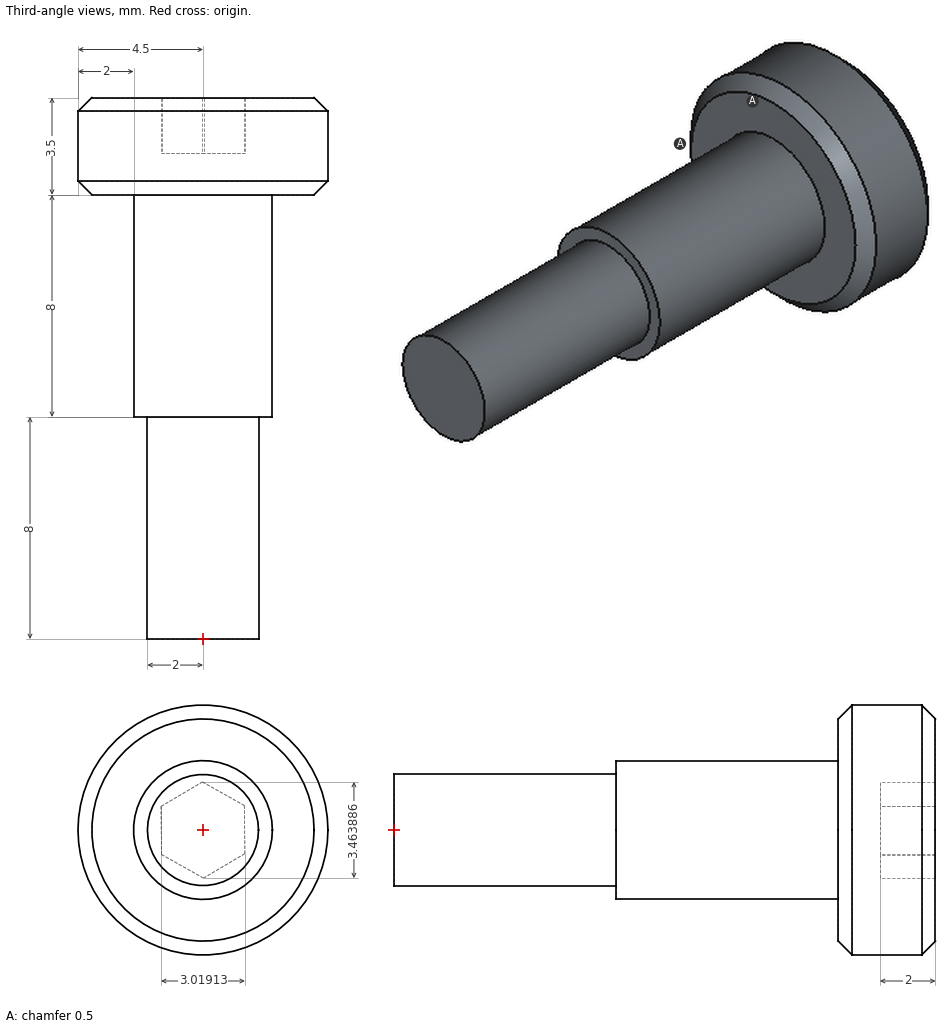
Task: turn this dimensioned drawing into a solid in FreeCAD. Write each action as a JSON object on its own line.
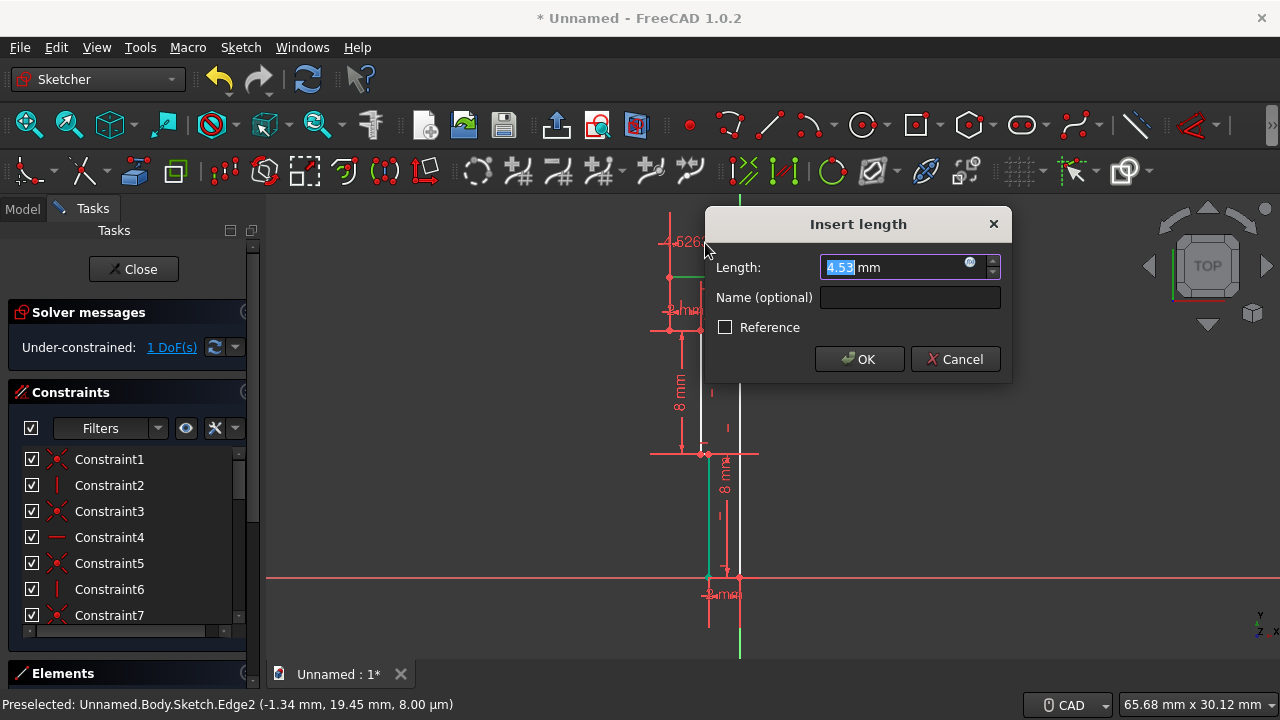
{"action": "type", "text": "4.5"}
{"action": "key", "text": "Return"}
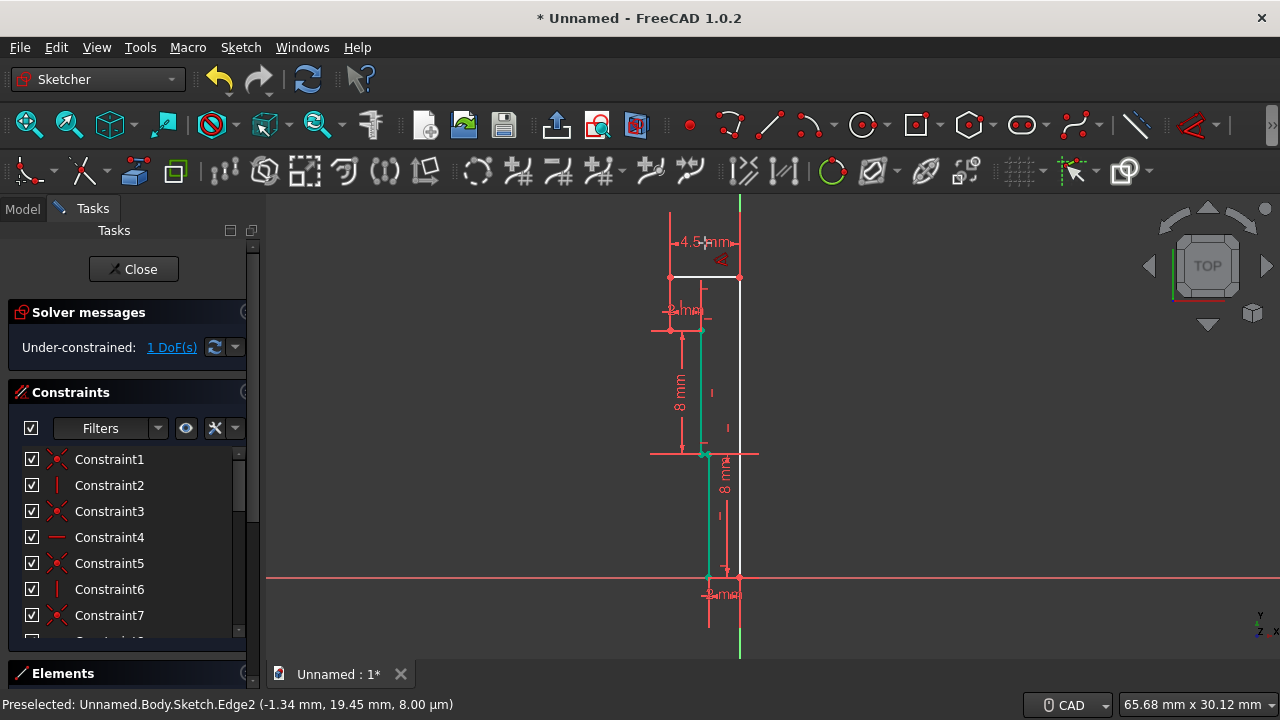
{"action": "left_click", "coordinate": [670, 293]}
{"action": "left_click", "coordinate": [636, 292]}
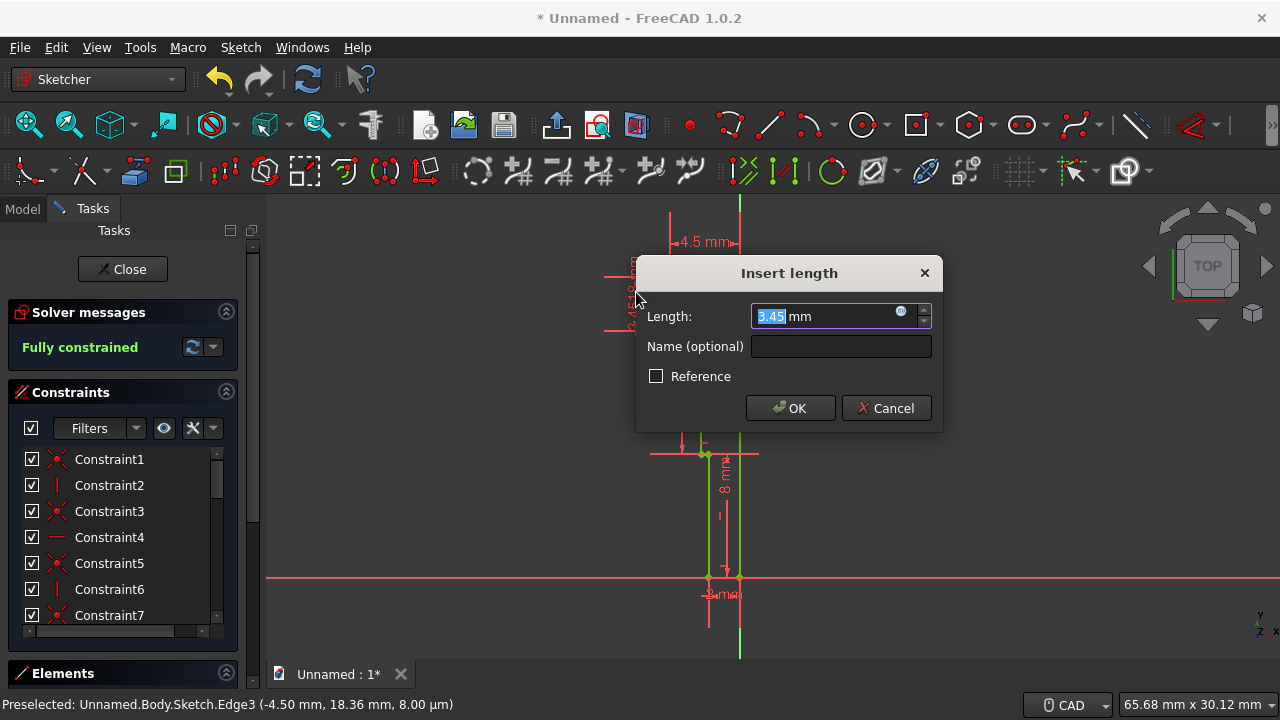
{"action": "type", "text": "3.5"}
{"action": "key", "text": "Return"}
{"action": "key", "text": "Escape"}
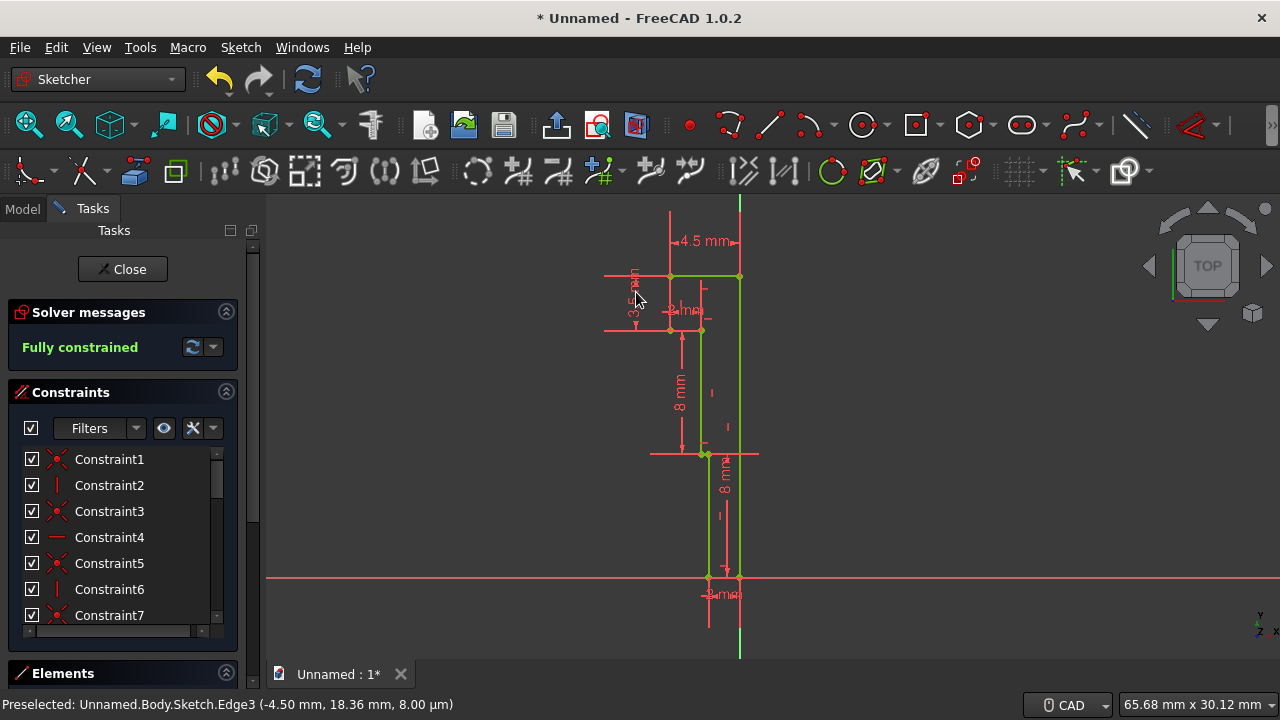
{"action": "left_click", "coordinate": [123, 269]}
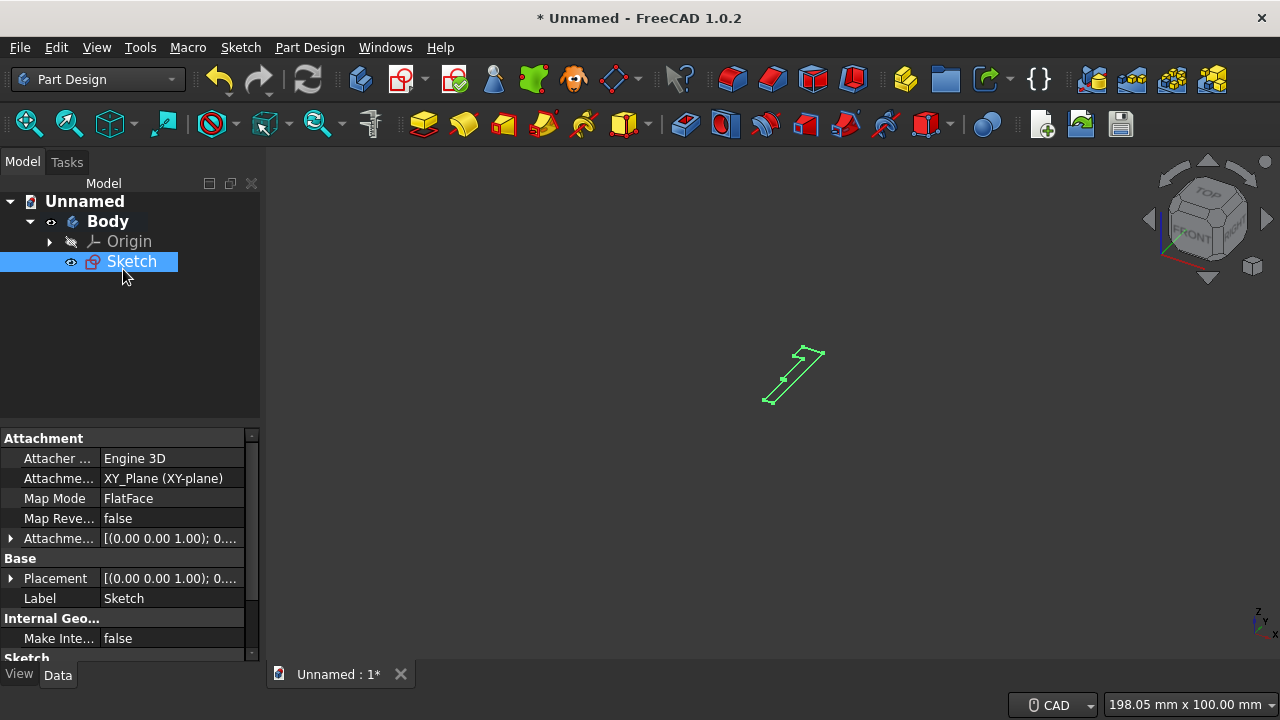
{"action": "left_click", "coordinate": [464, 124]}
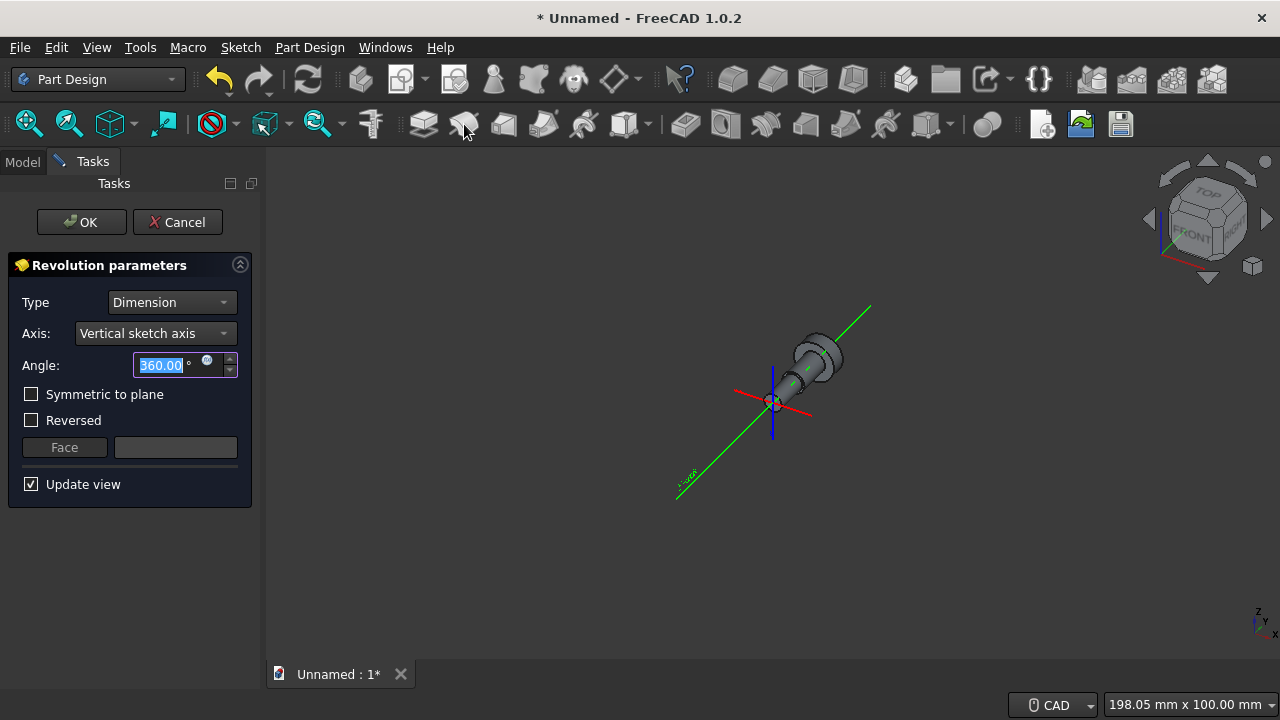
{"action": "left_click", "coordinate": [82, 222]}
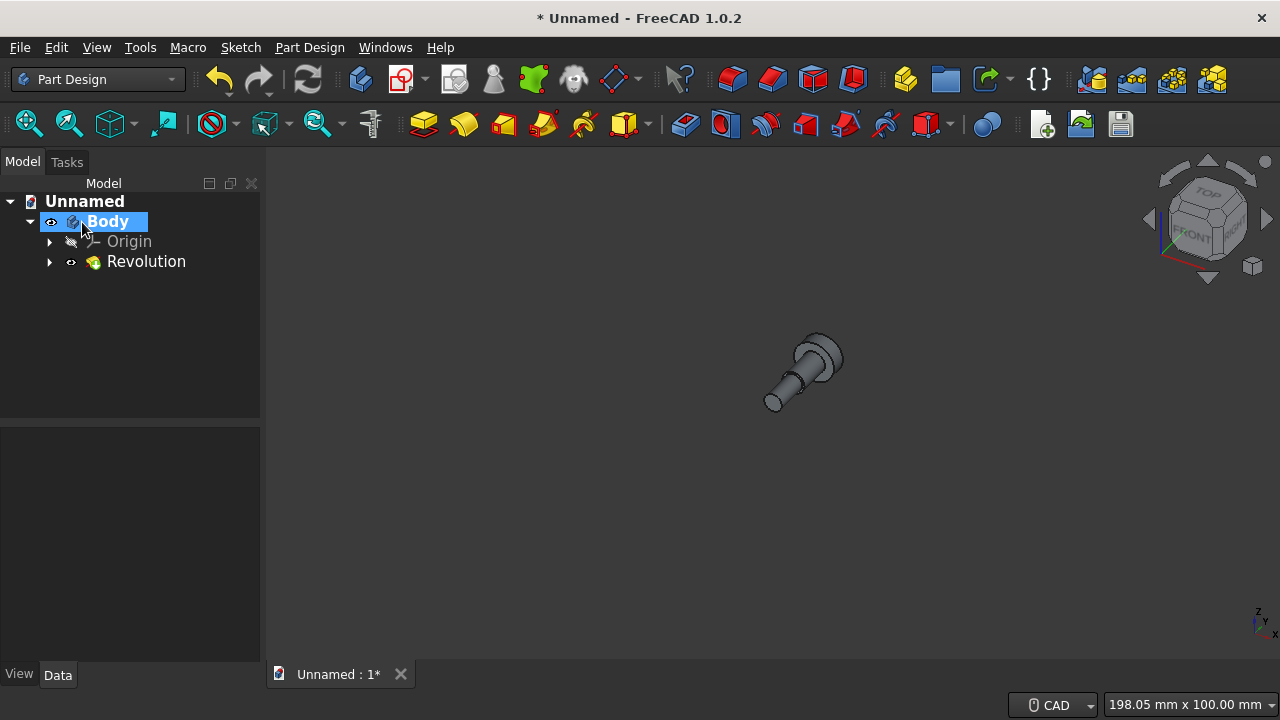
{"action": "key", "text": "v f"}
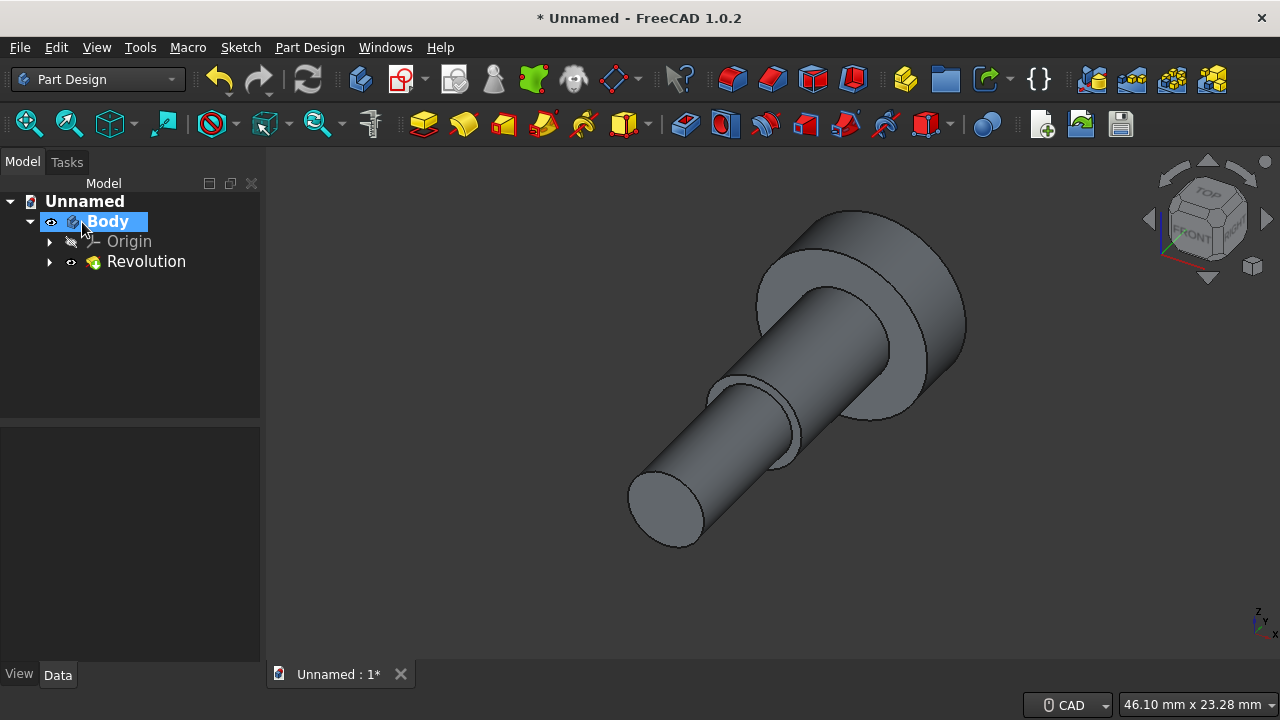
{"action": "key", "text": "4"}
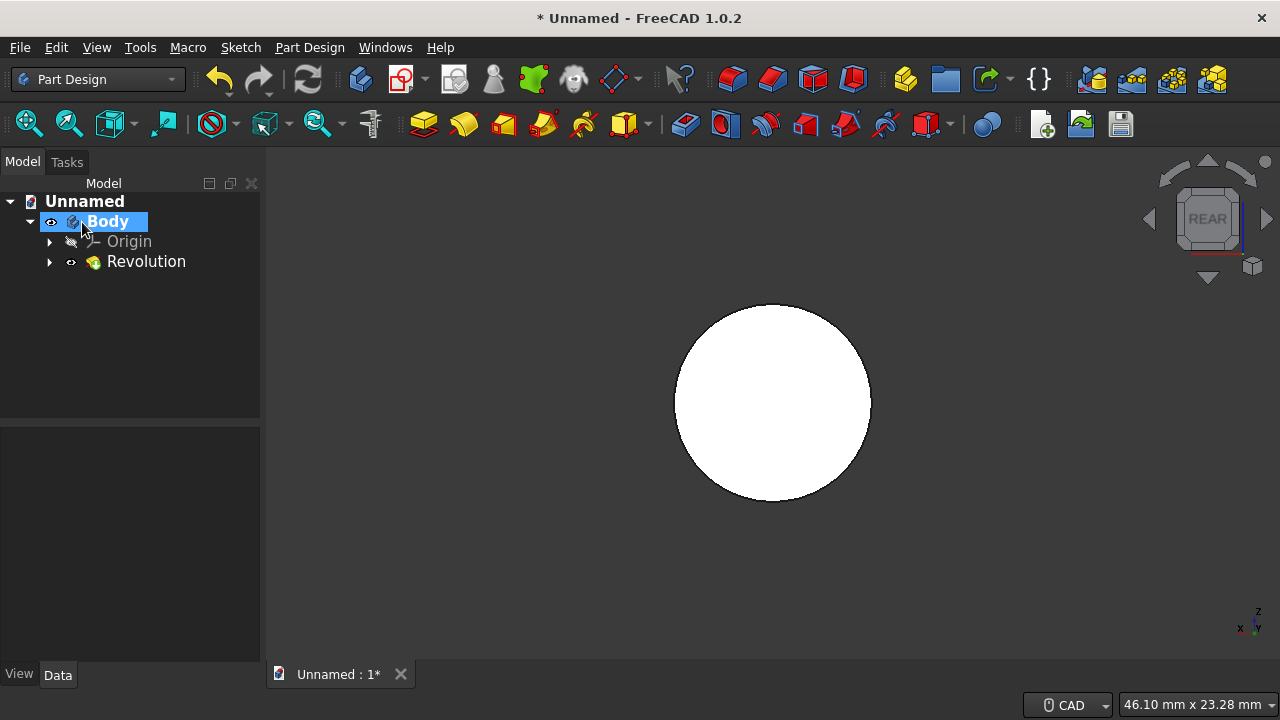
{"action": "left_click", "coordinate": [30, 124]}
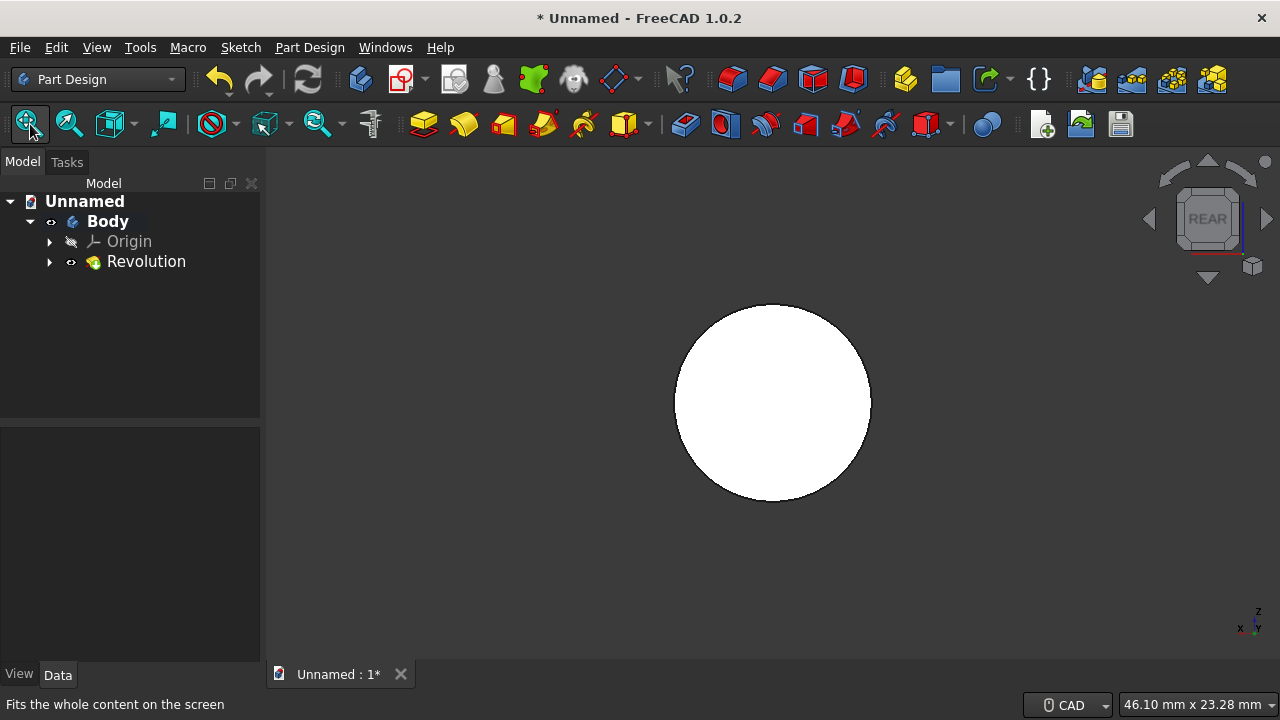
{"action": "left_click", "coordinate": [773, 402]}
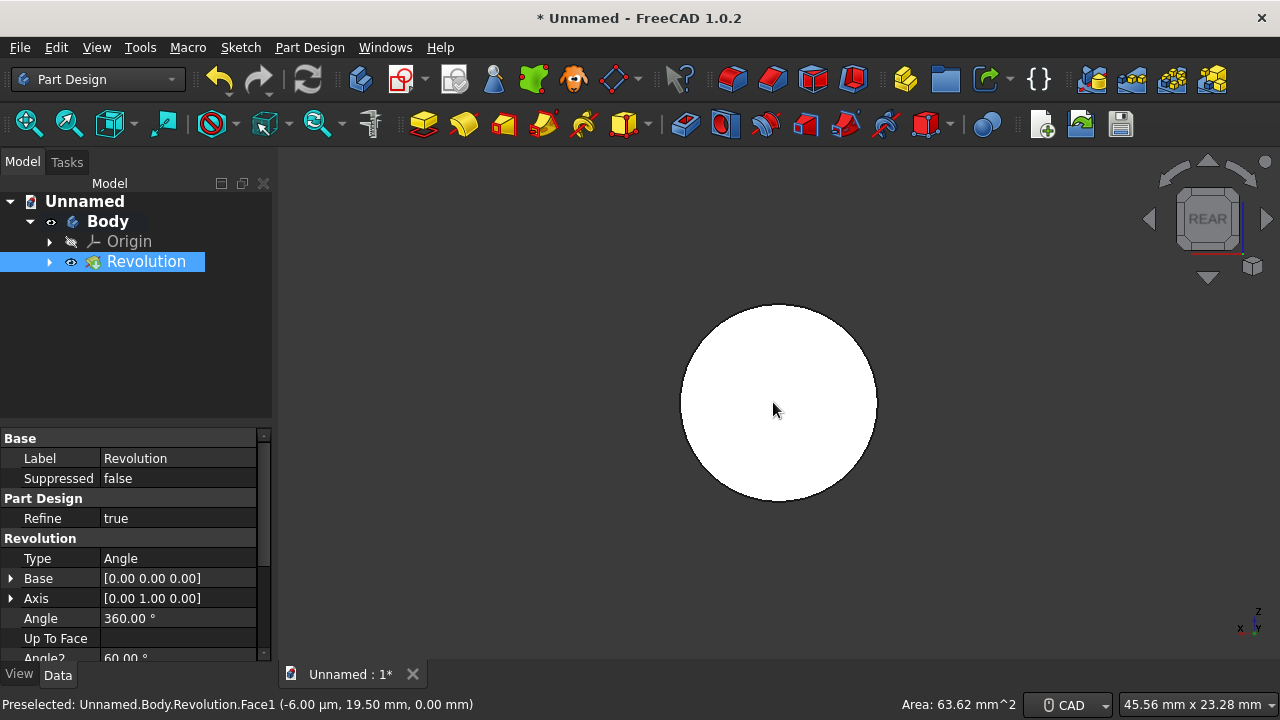
{"action": "left_click", "coordinate": [402, 80]}